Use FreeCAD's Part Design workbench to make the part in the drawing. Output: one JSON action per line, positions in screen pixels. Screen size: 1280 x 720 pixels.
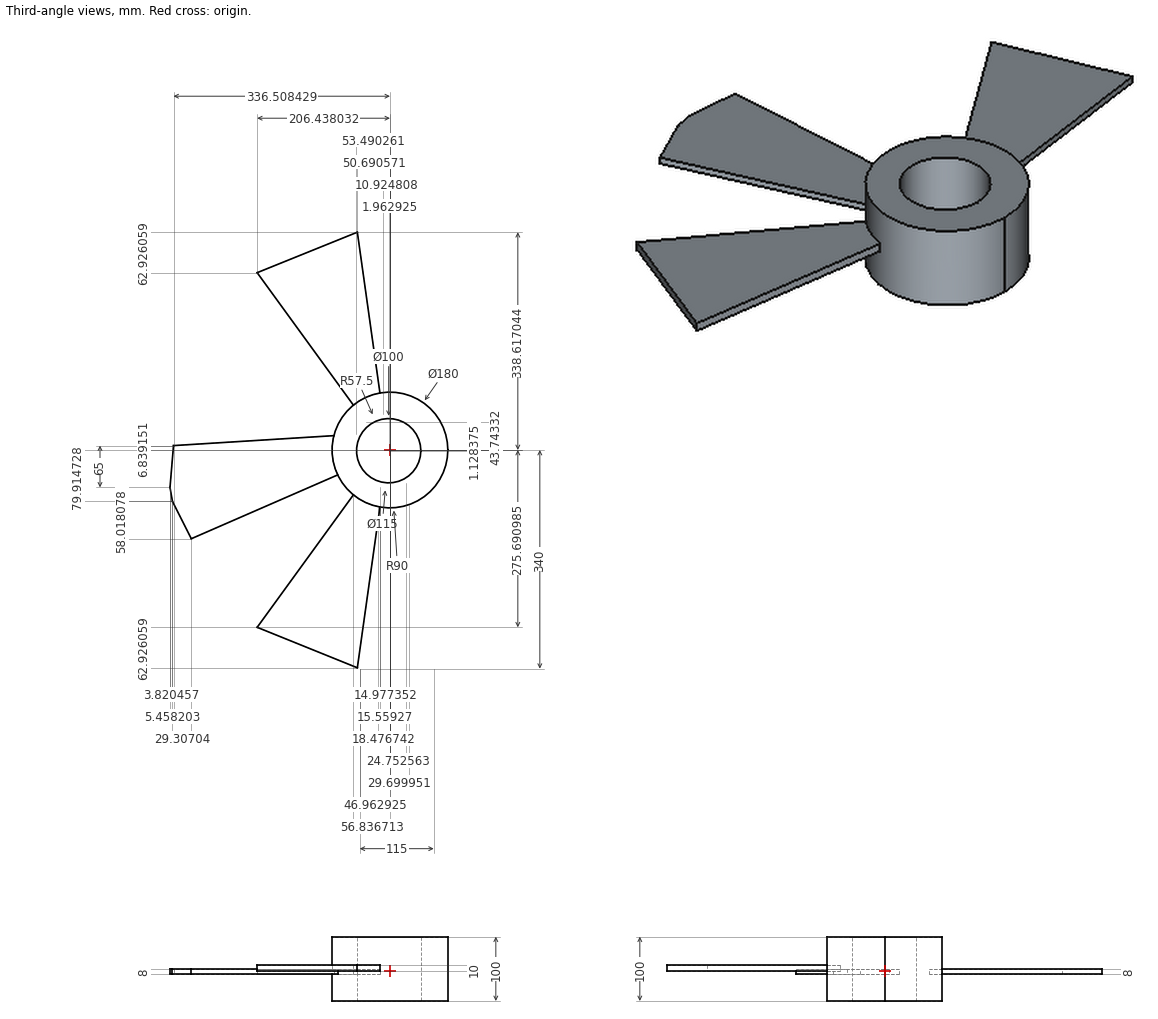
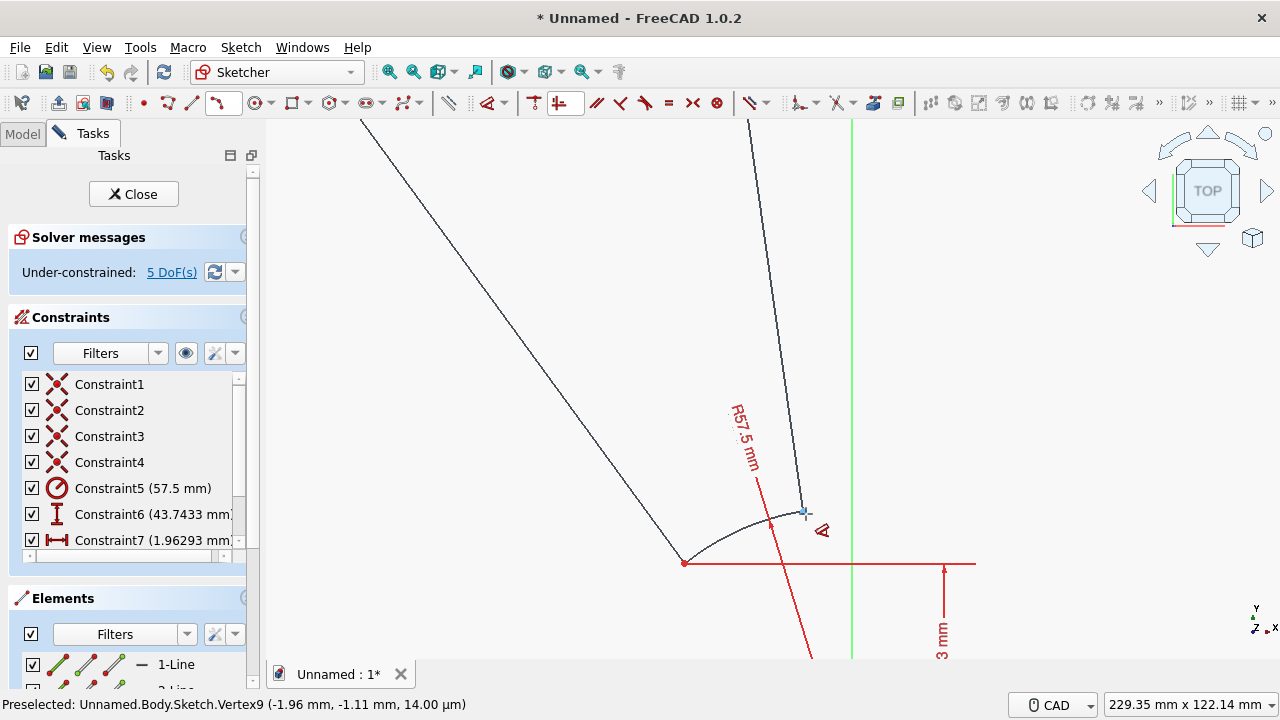
{"action": "left_click", "coordinate": [803, 511]}
{"action": "left_click", "coordinate": [828, 477]}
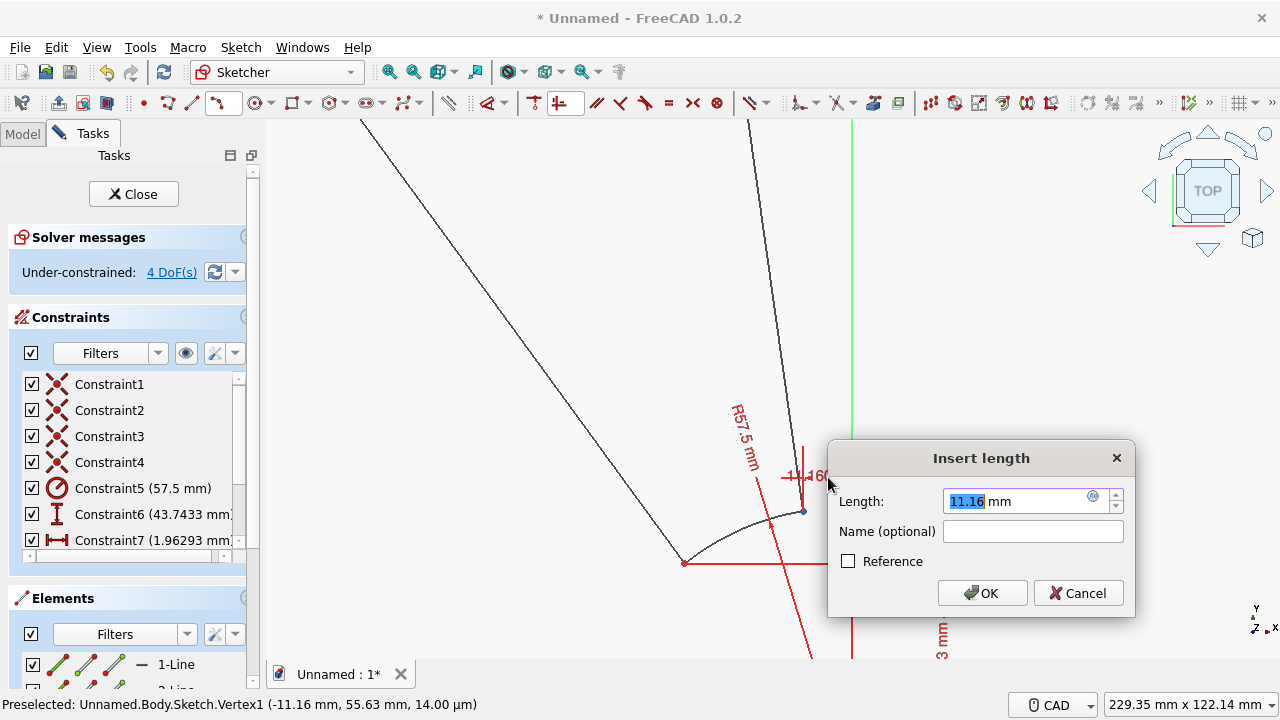
{"action": "type", "text": "10.924808"}
{"action": "key", "text": "Return"}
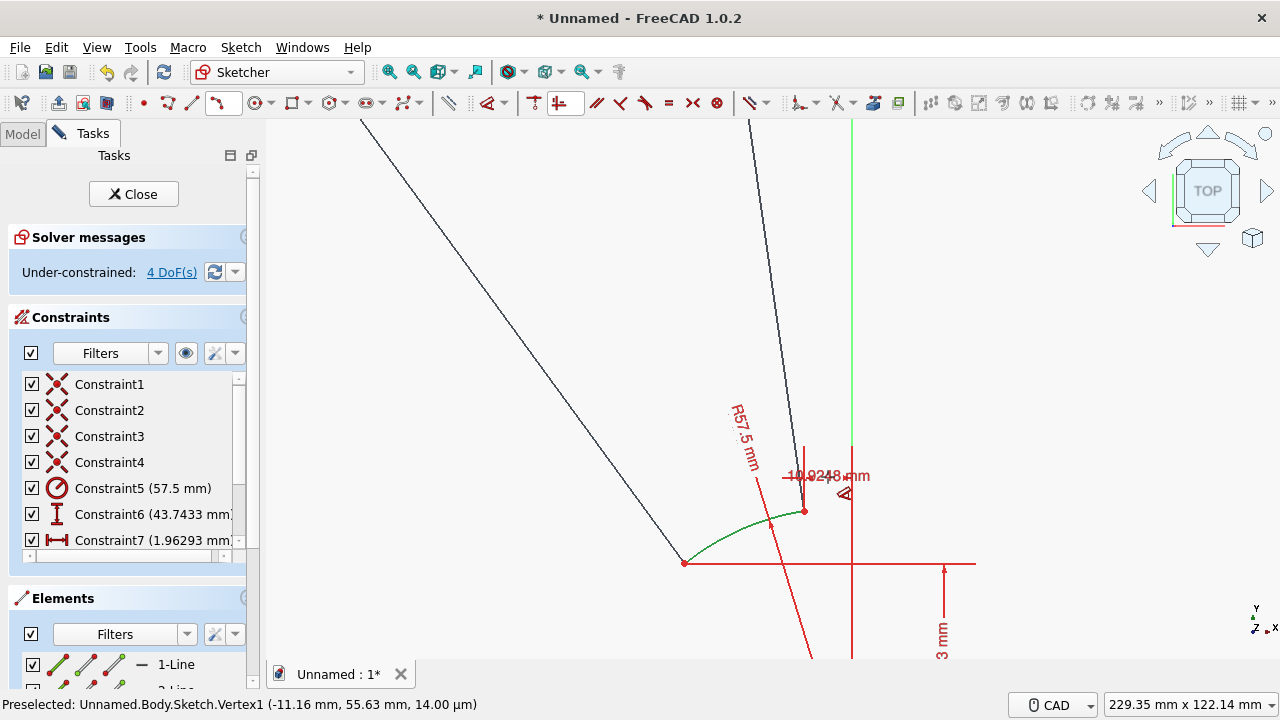
{"action": "scroll", "coordinate": [805, 514], "scroll_direction": "down", "scroll_amount": 7}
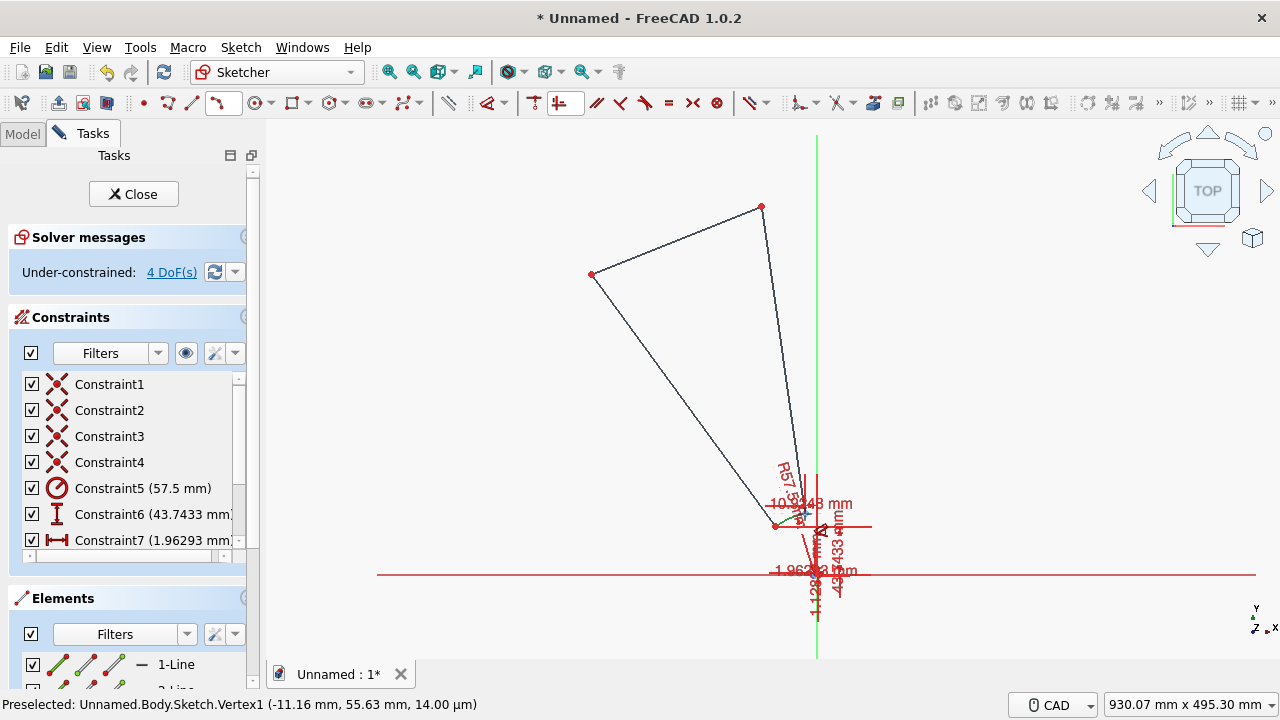
{"action": "left_click", "coordinate": [762, 207]}
{"action": "left_click", "coordinate": [789, 609]}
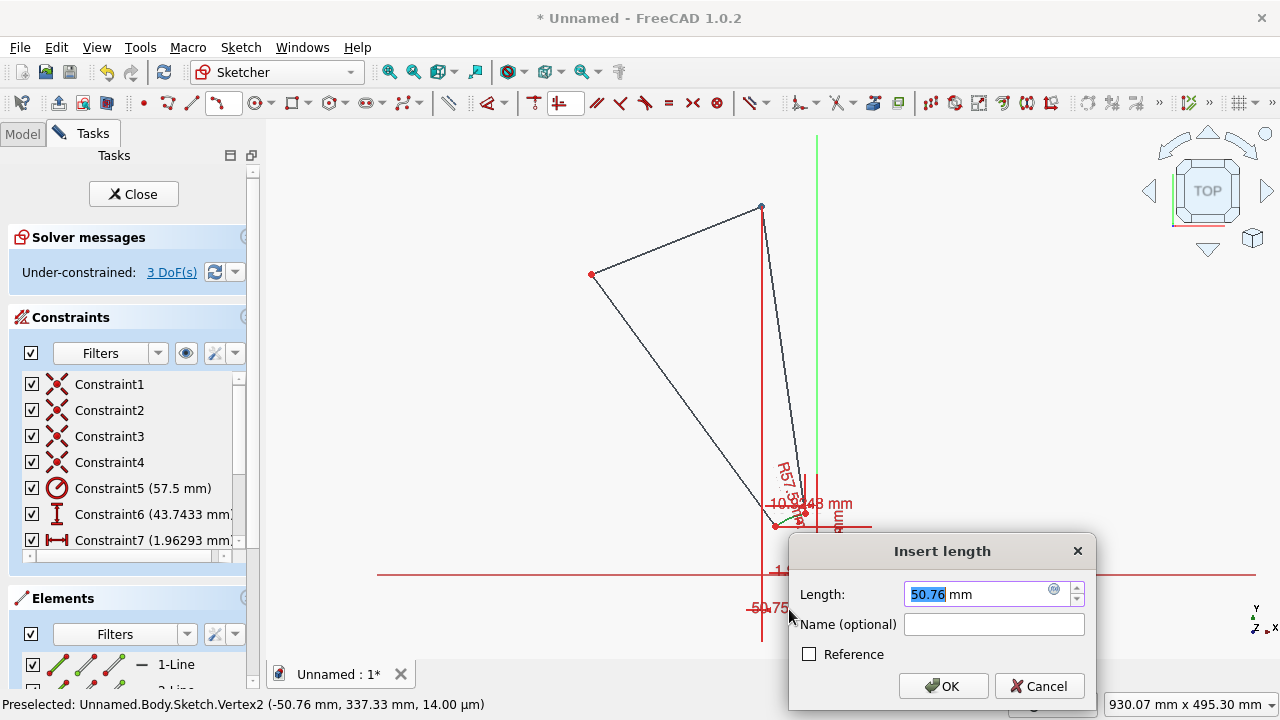
{"action": "type", "text": "50.690571"}
{"action": "key", "text": "Return"}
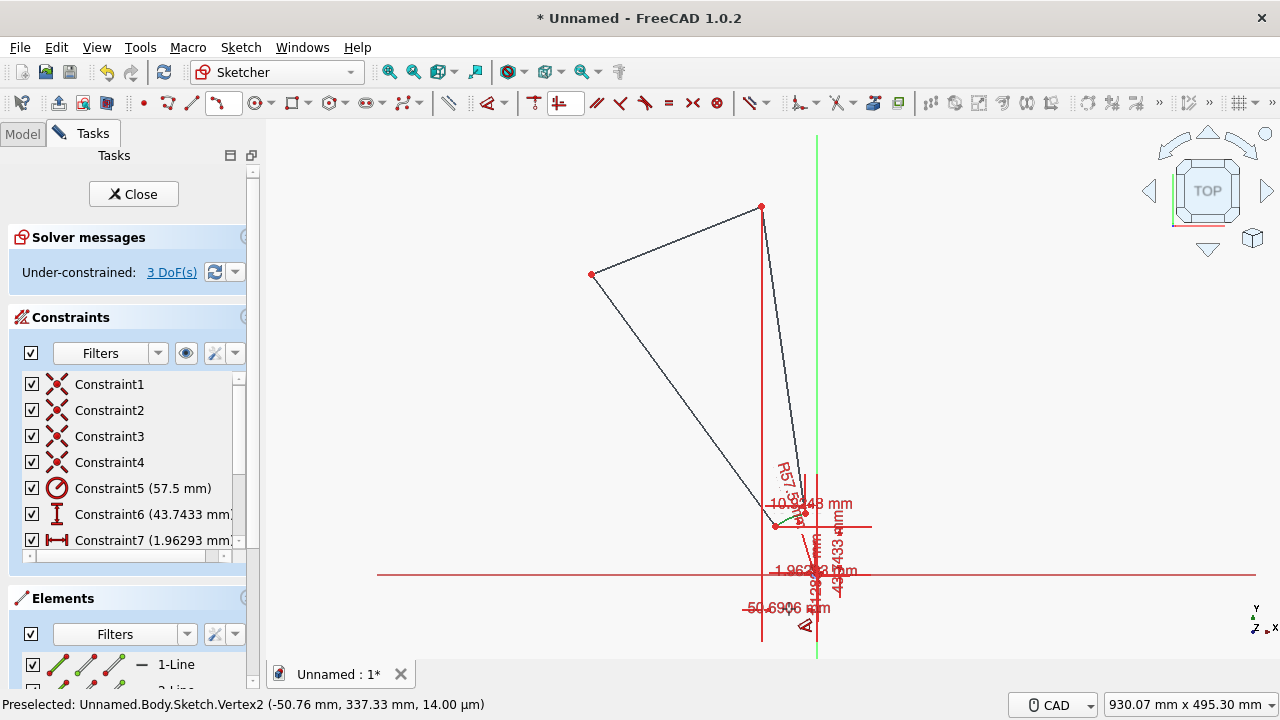
{"action": "left_click", "coordinate": [711, 227]}
{"action": "left_click", "coordinate": [558, 241]}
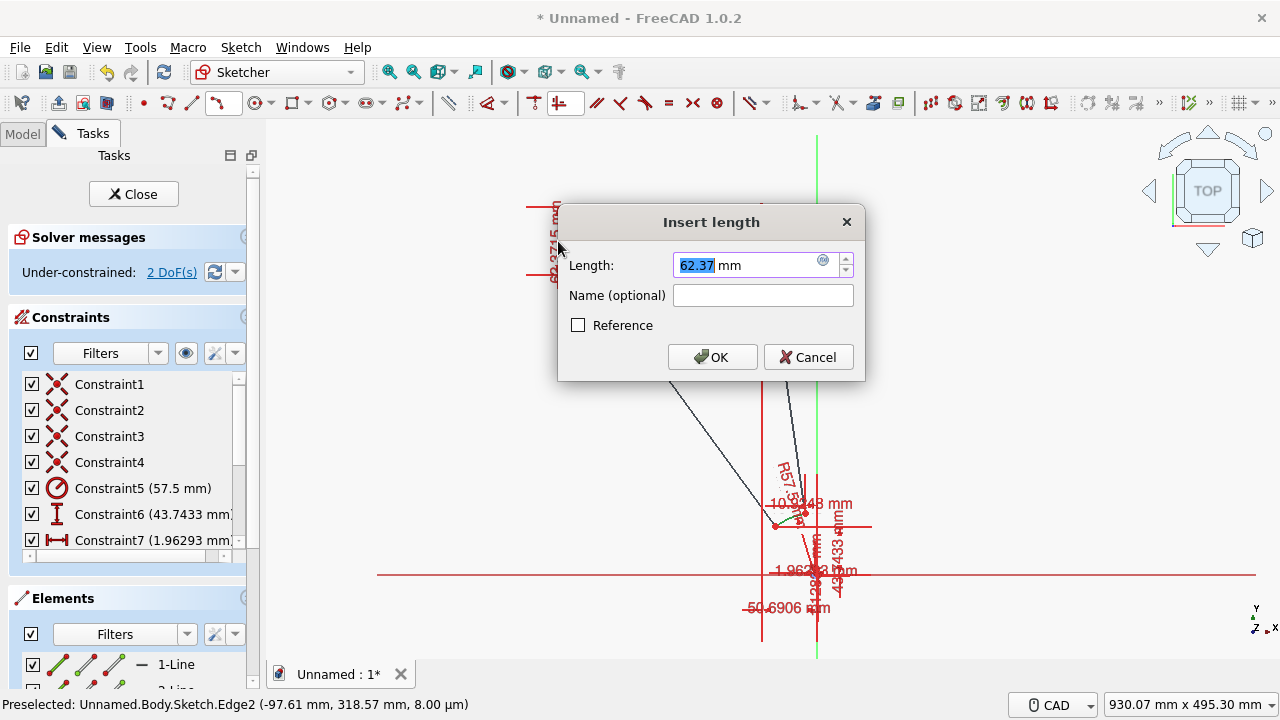
{"action": "type", "text": "62.926059"}
{"action": "key", "text": "Return"}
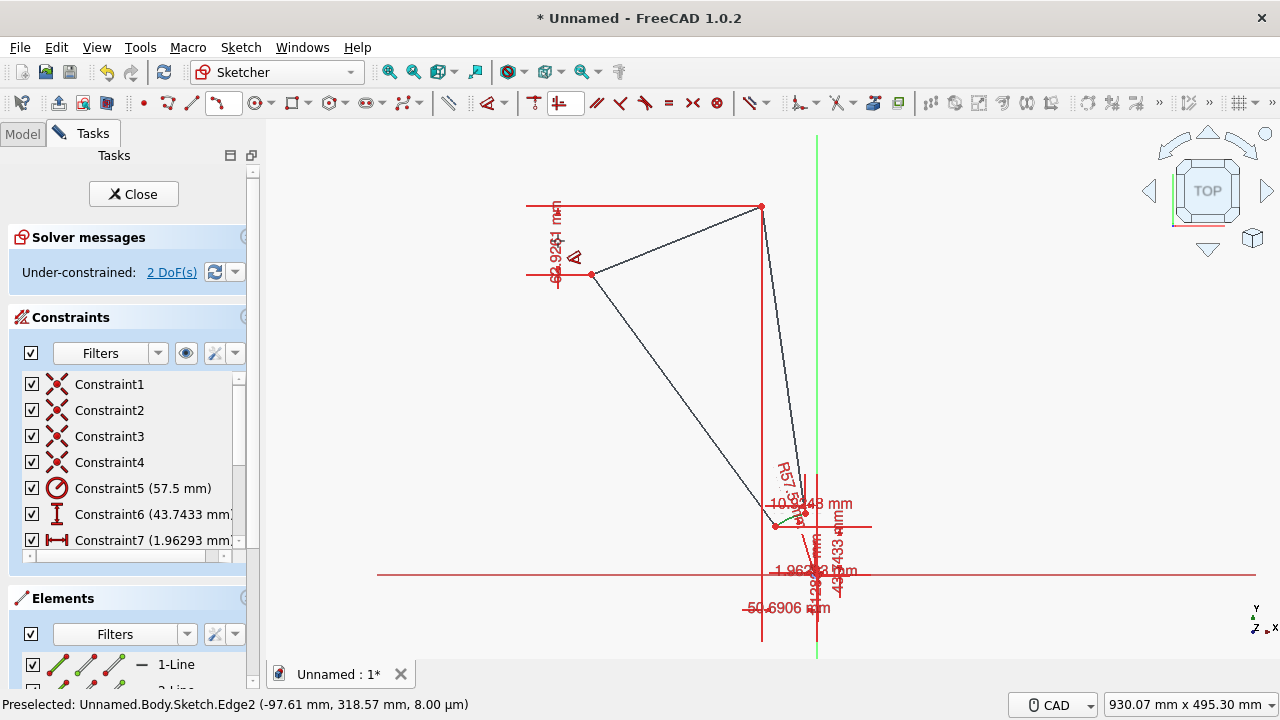
{"action": "left_click", "coordinate": [762, 206]}
{"action": "left_click", "coordinate": [851, 390]}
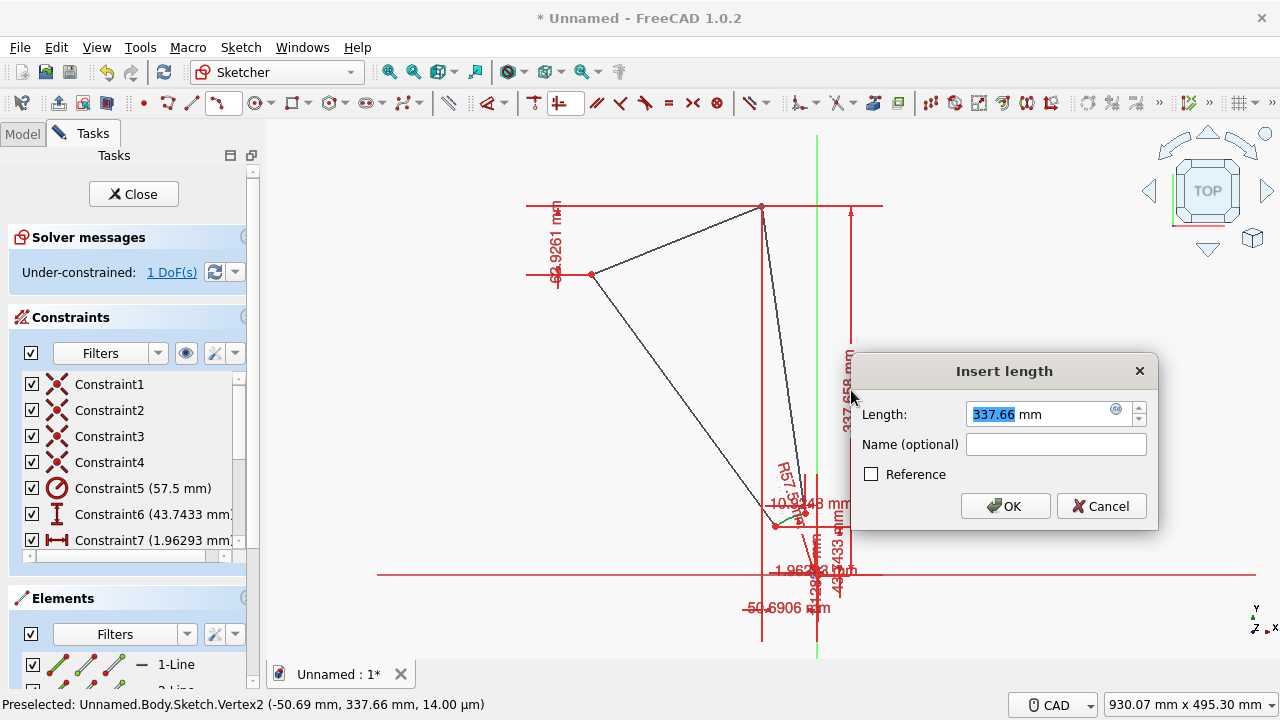
{"action": "type", "text": "338.617044"}
{"action": "key", "text": "Return"}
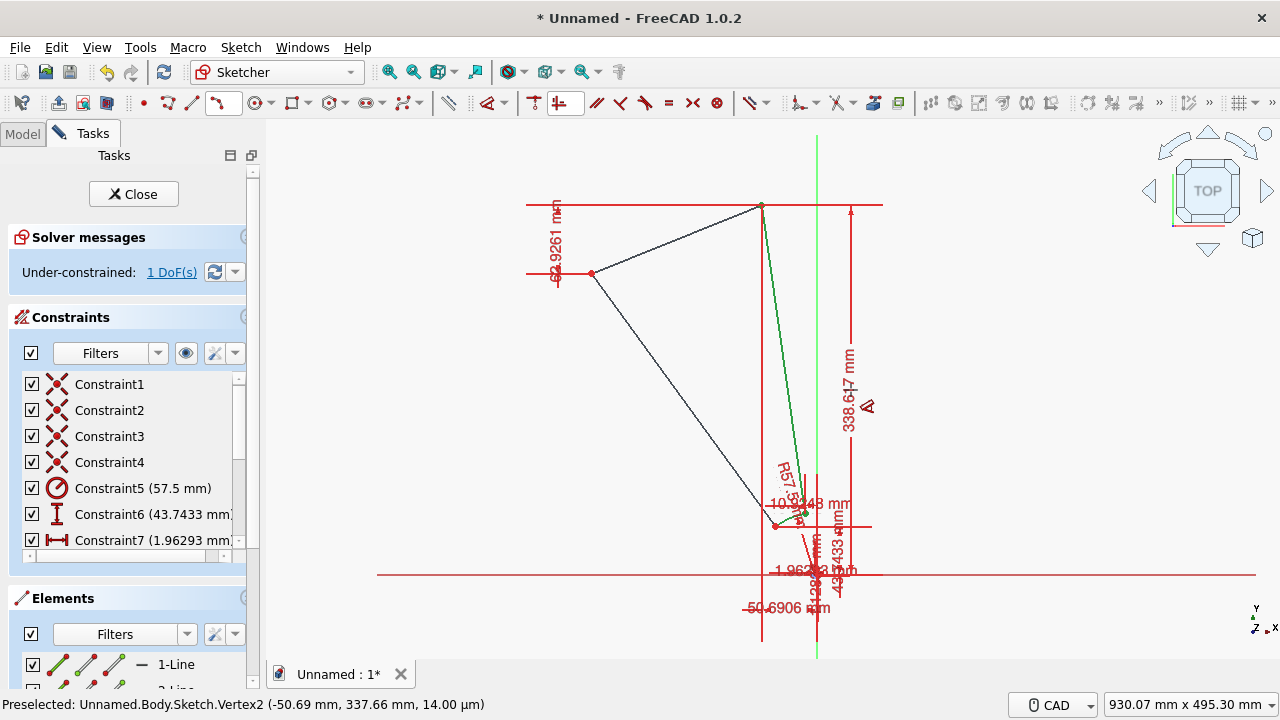
{"action": "left_click", "coordinate": [592, 274]}
{"action": "left_click", "coordinate": [704, 609]}